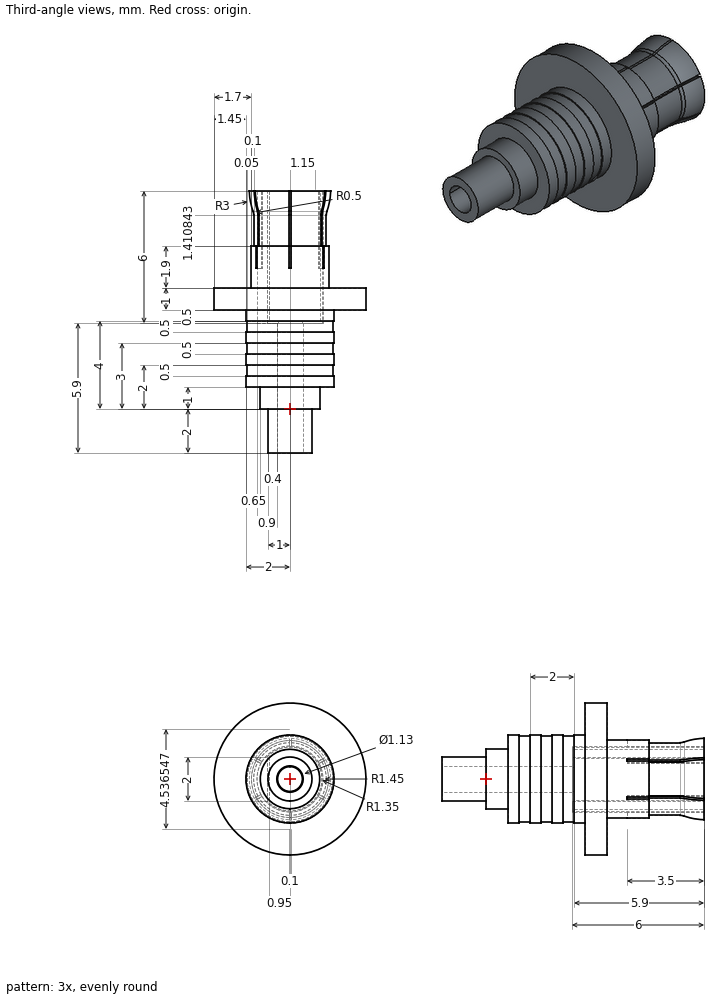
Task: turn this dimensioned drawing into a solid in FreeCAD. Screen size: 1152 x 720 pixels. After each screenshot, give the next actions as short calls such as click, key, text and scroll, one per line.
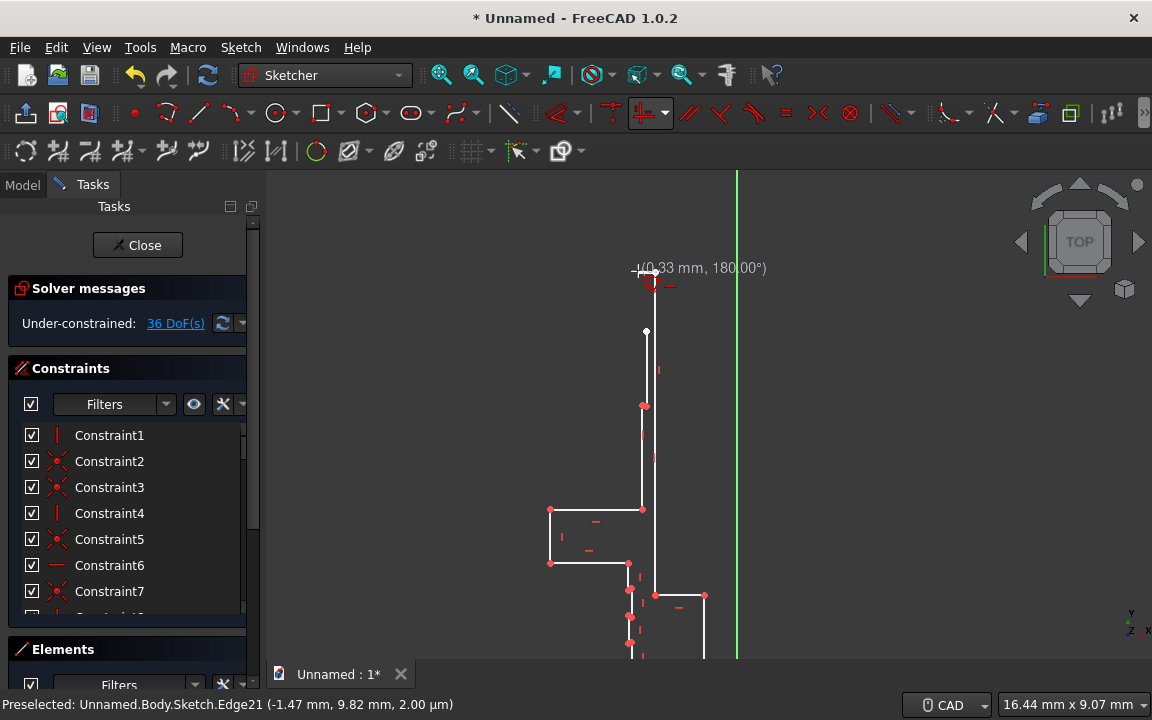
click(637, 271)
right_click(637, 271)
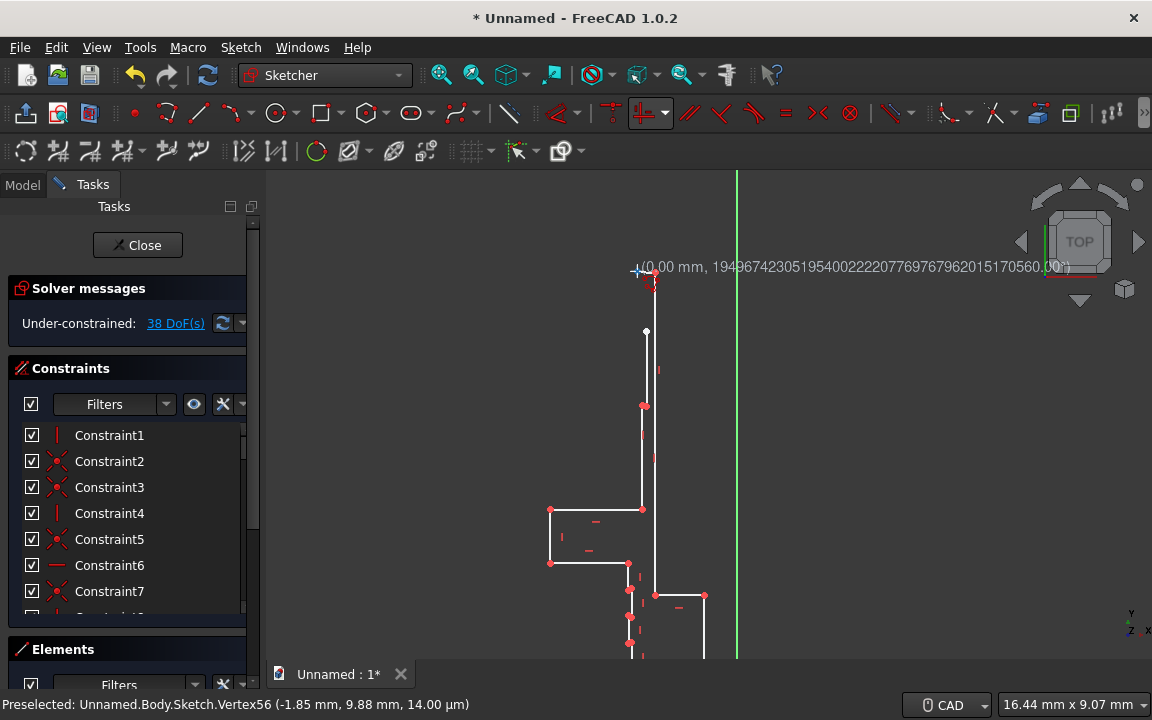
click(232, 114)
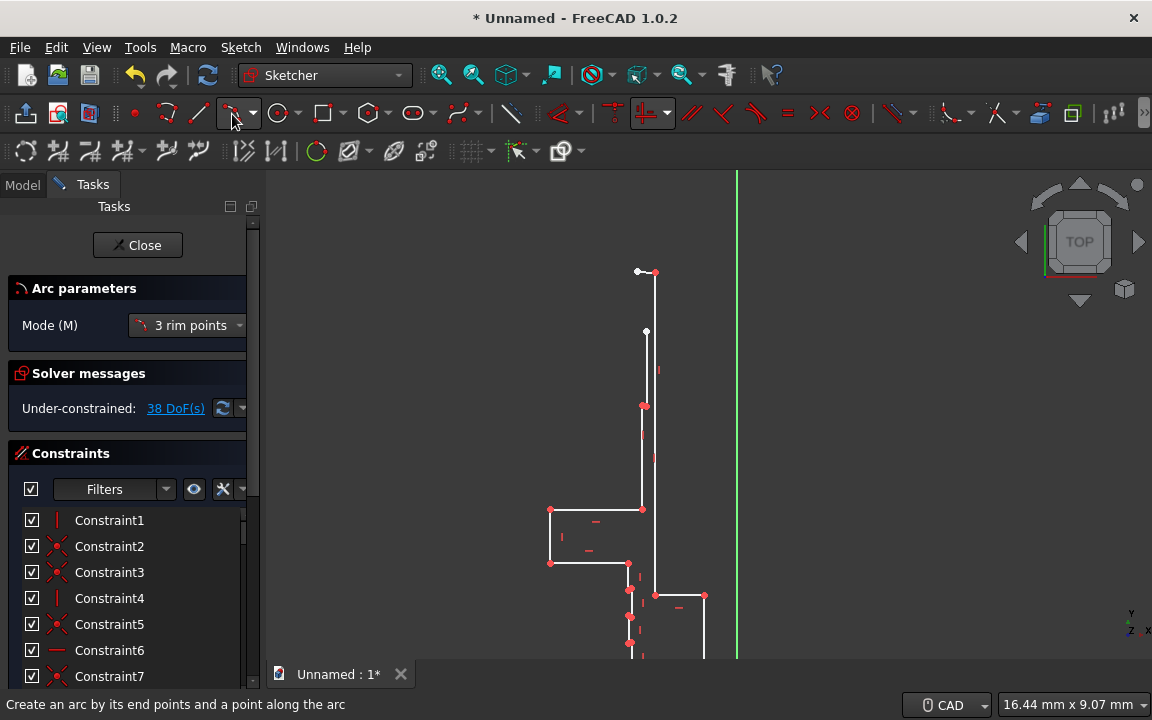
scroll(637, 271, up, 3)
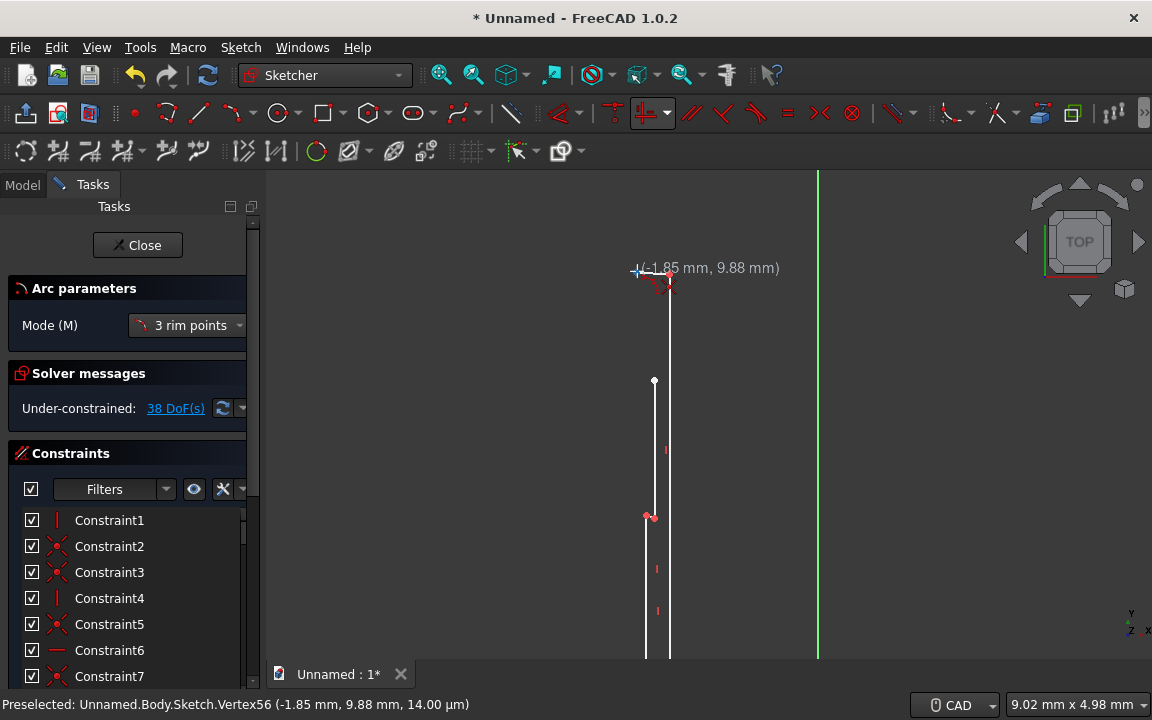
click(637, 273)
click(653, 361)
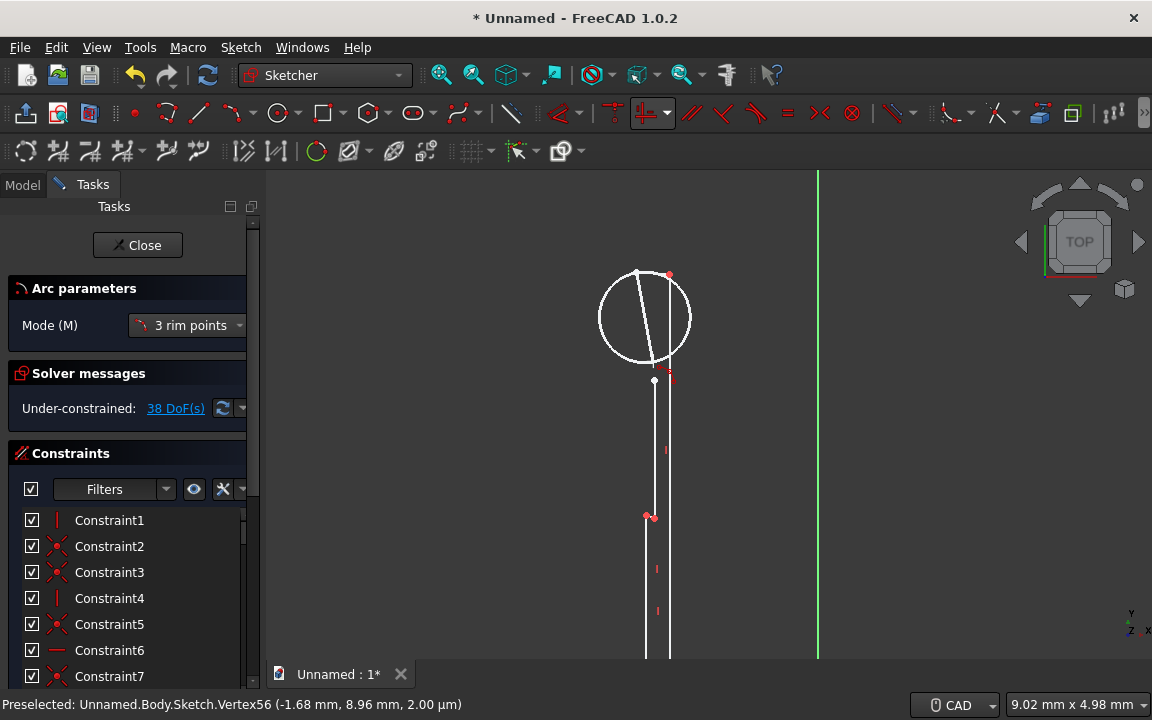
scroll(641, 316, up, 8)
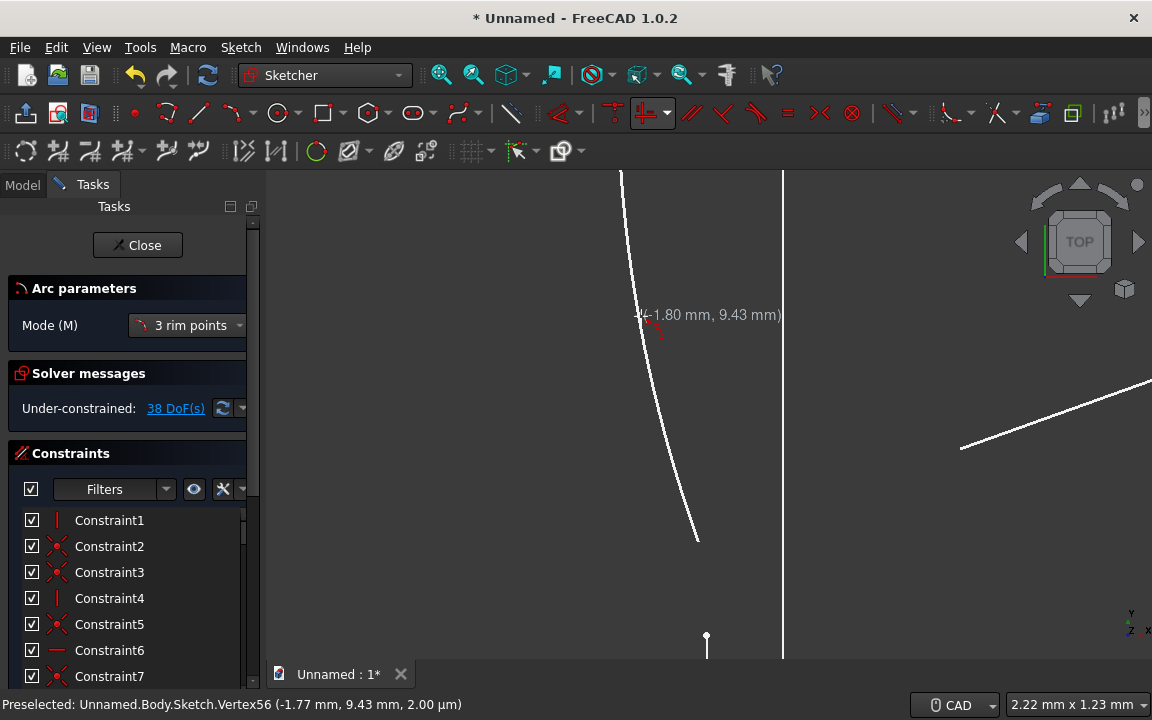
click(641, 317)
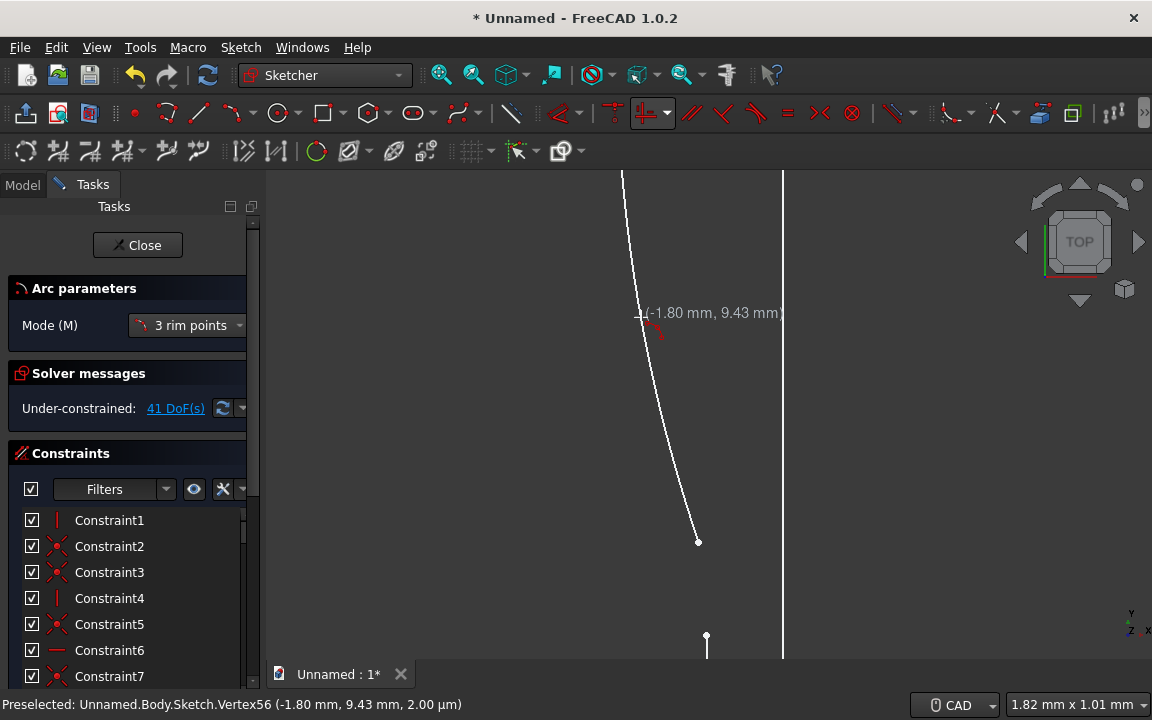
scroll(639, 280, down, 15)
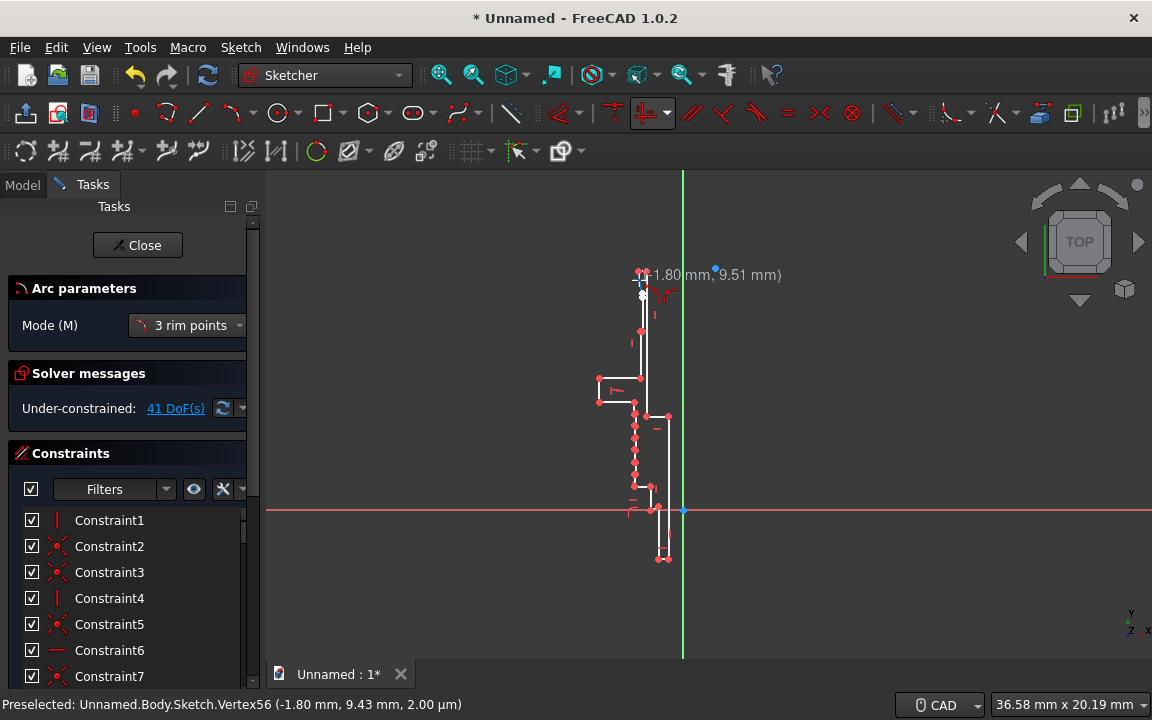
scroll(642, 293, up, 7)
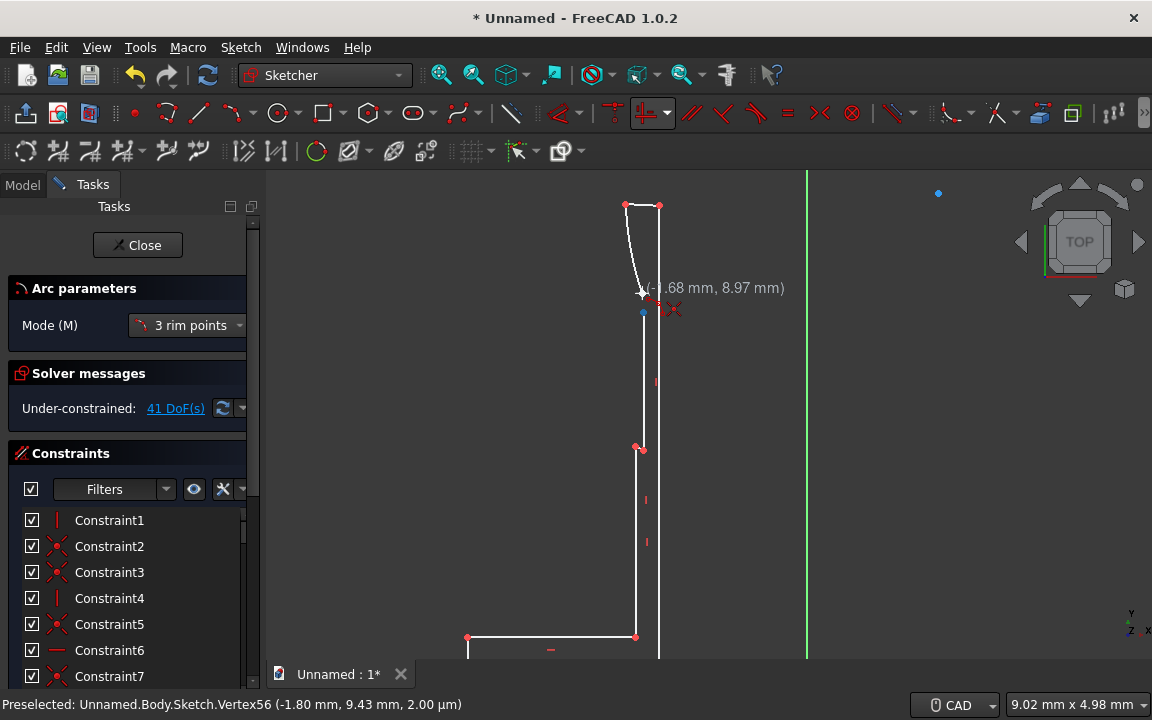
click(642, 293)
click(644, 312)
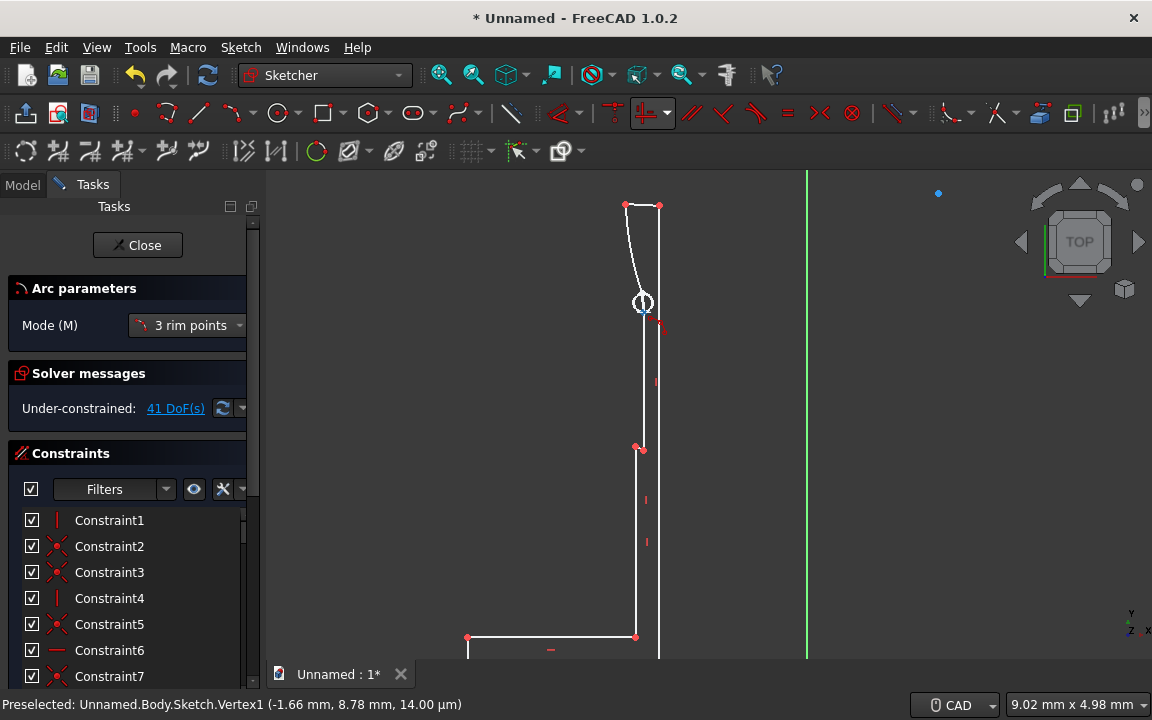
scroll(645, 300, up, 16)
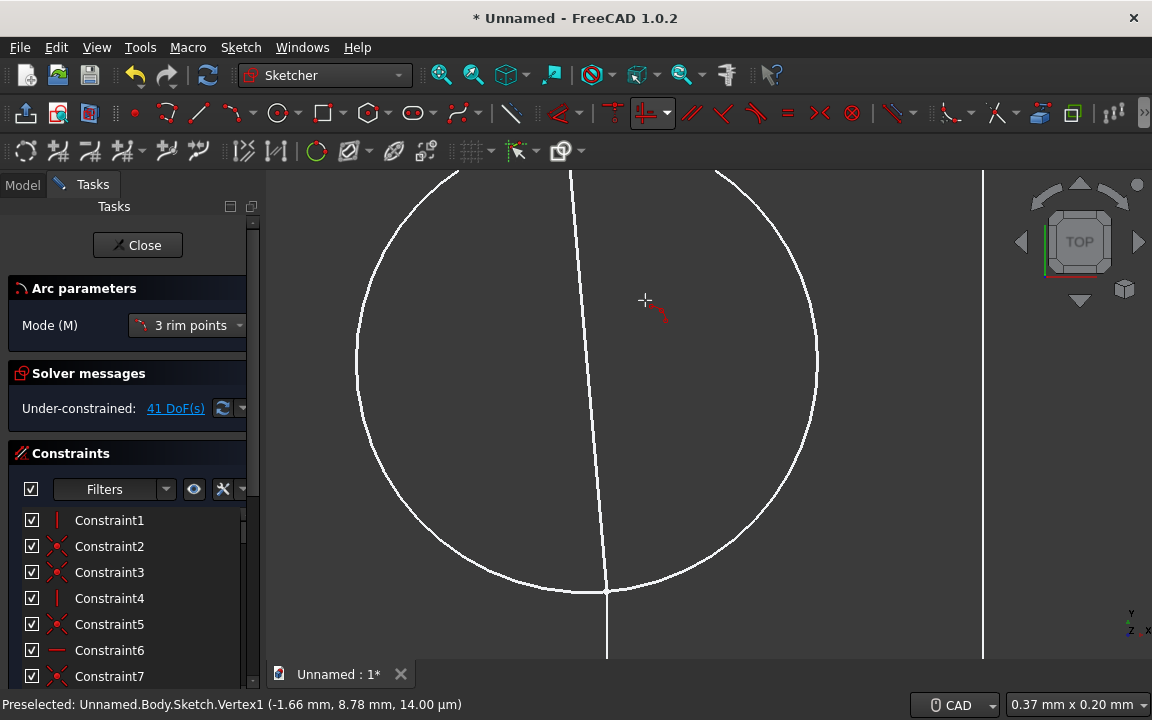
click(625, 305)
key(Escape)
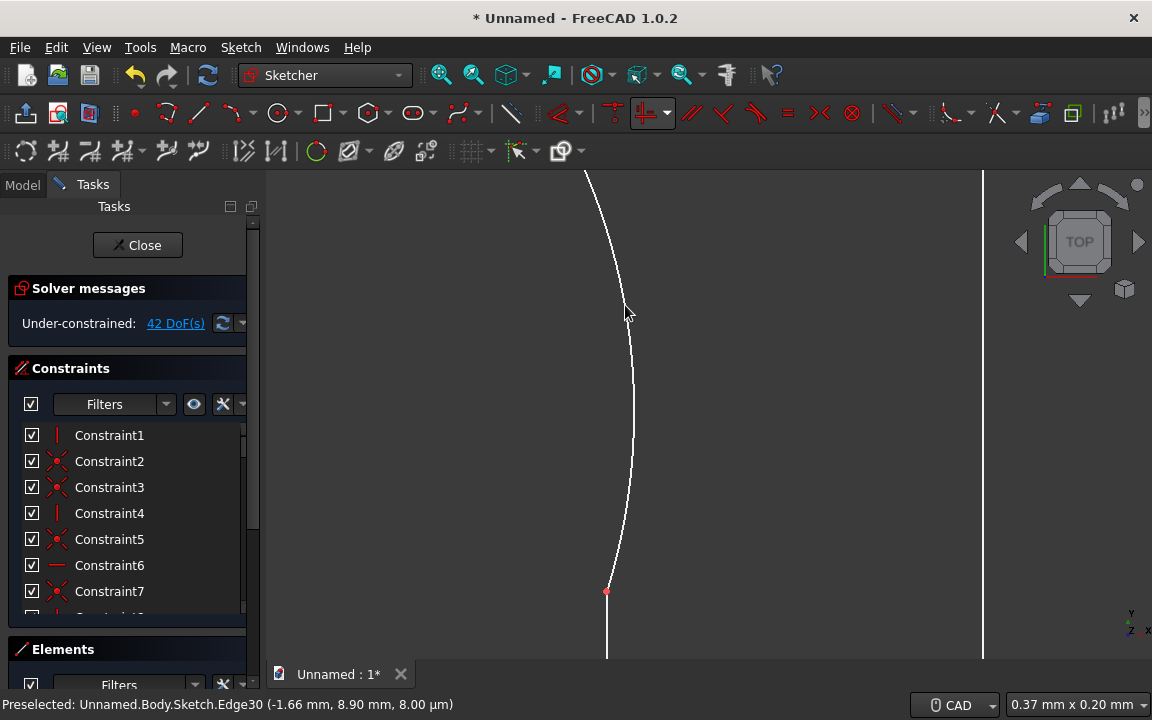
scroll(640, 414, down, 15)